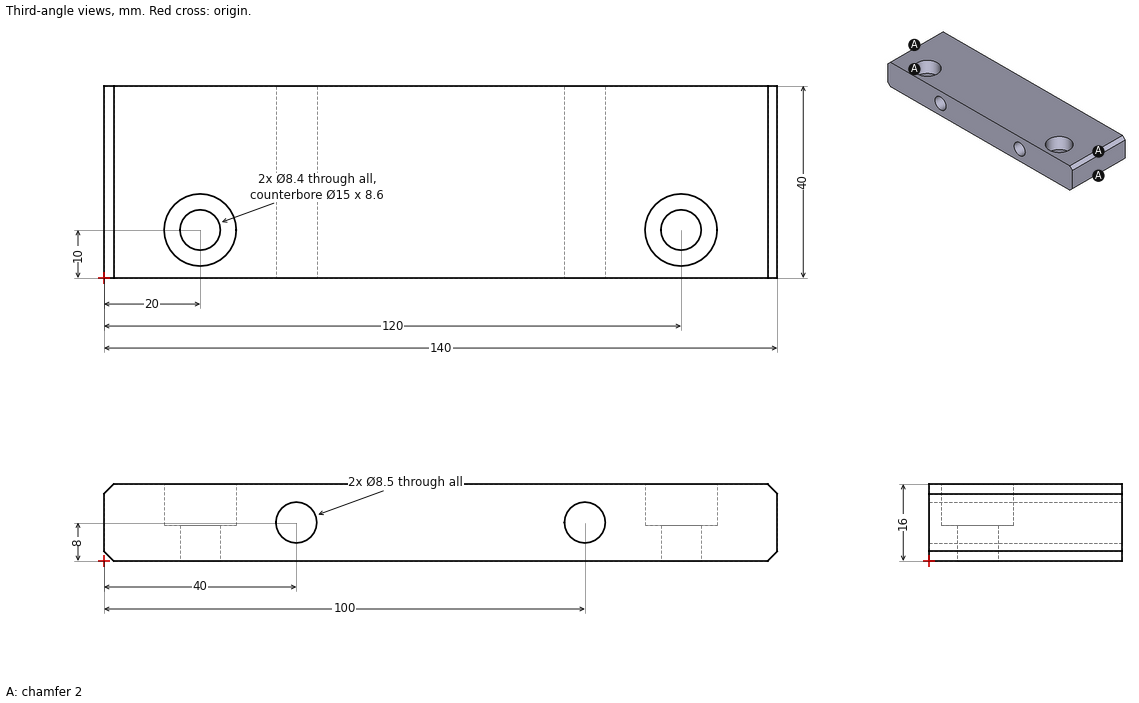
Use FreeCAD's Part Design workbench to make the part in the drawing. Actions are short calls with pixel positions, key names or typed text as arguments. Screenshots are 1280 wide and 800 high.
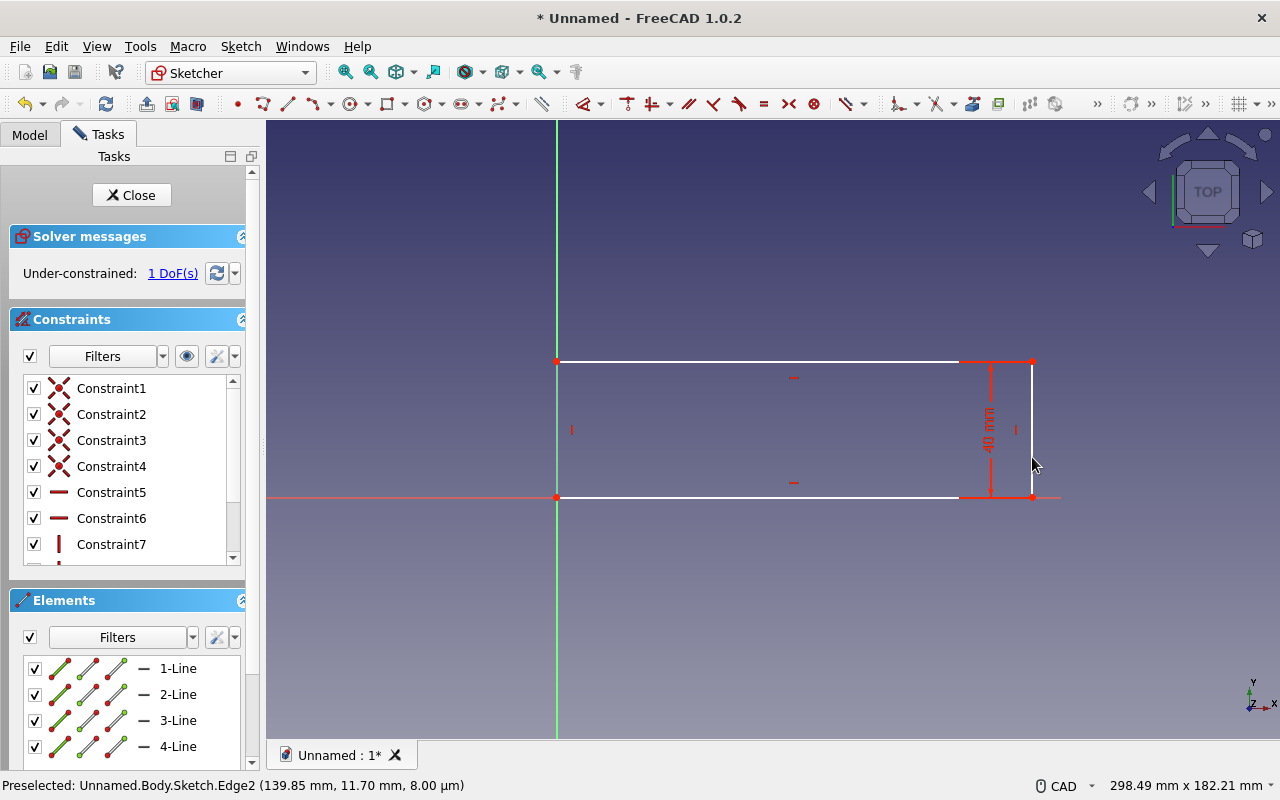
click(699, 498)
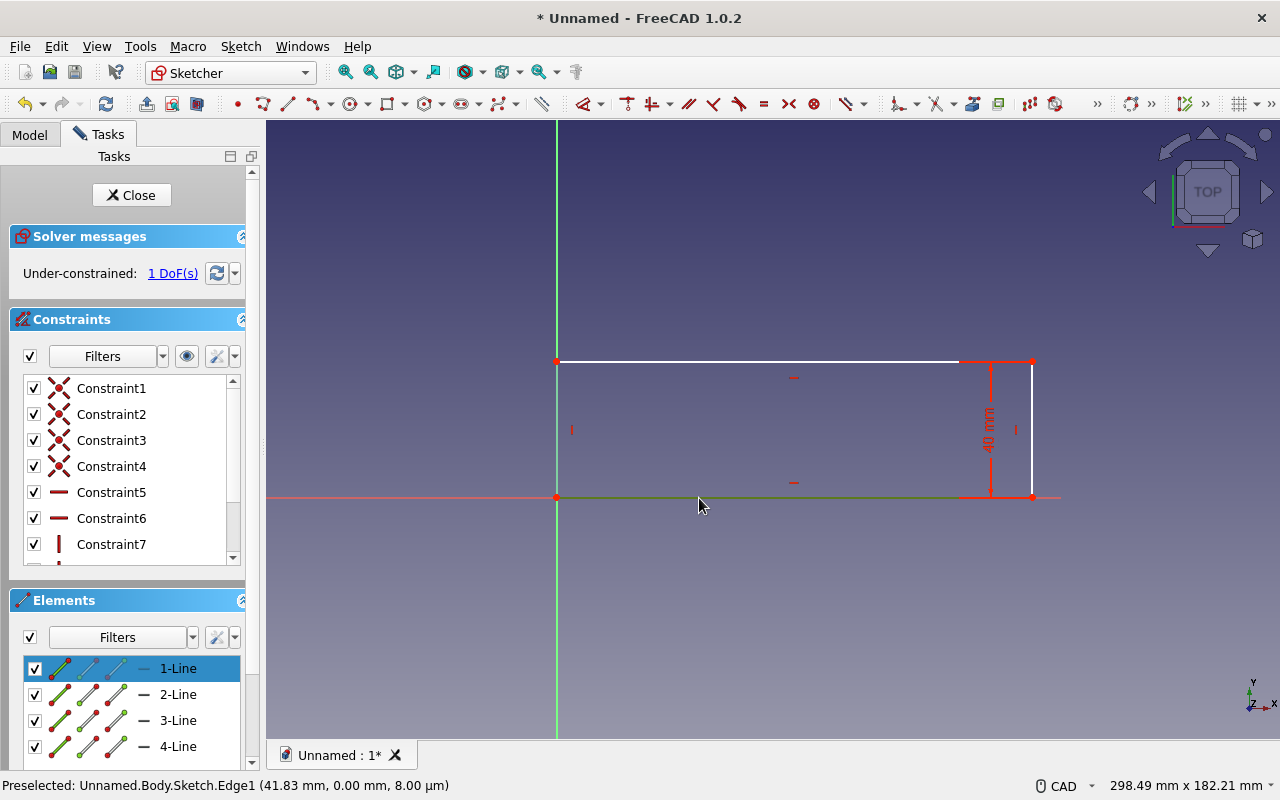
click(600, 104)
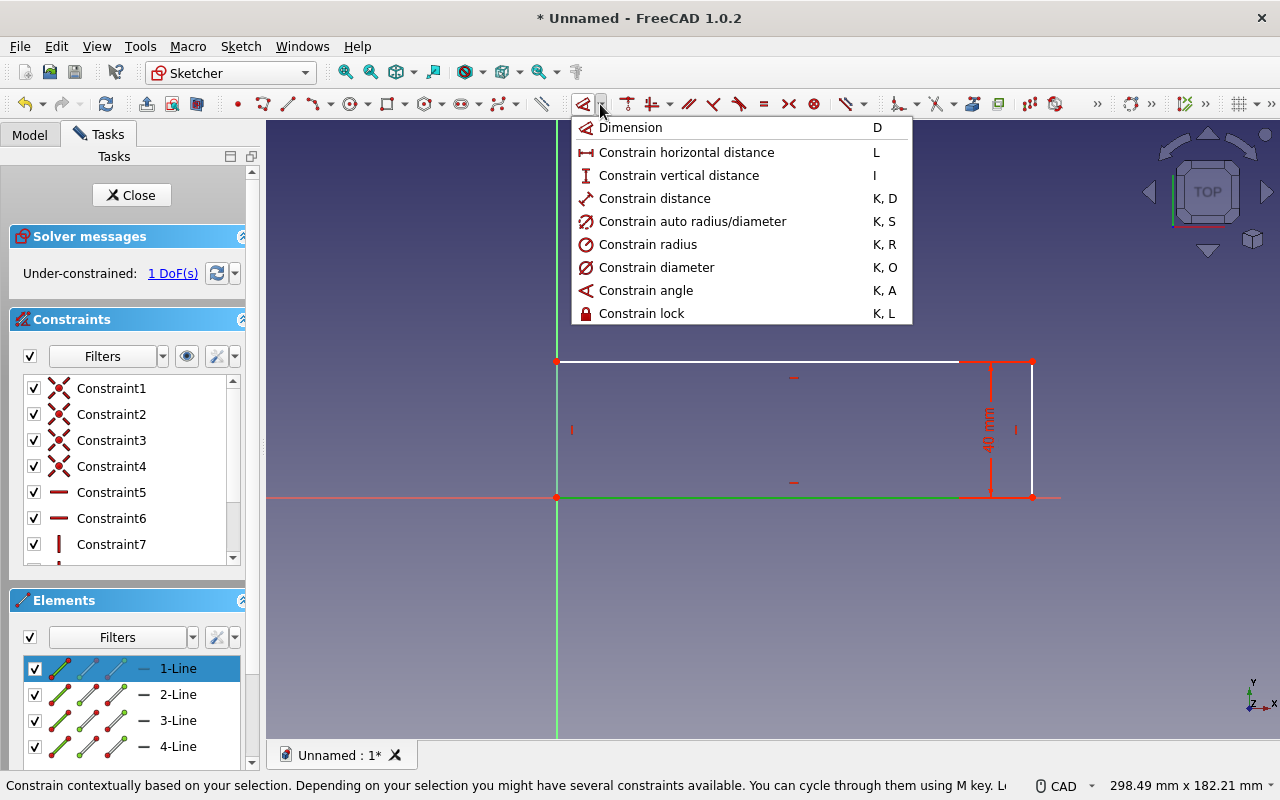
click(742, 152)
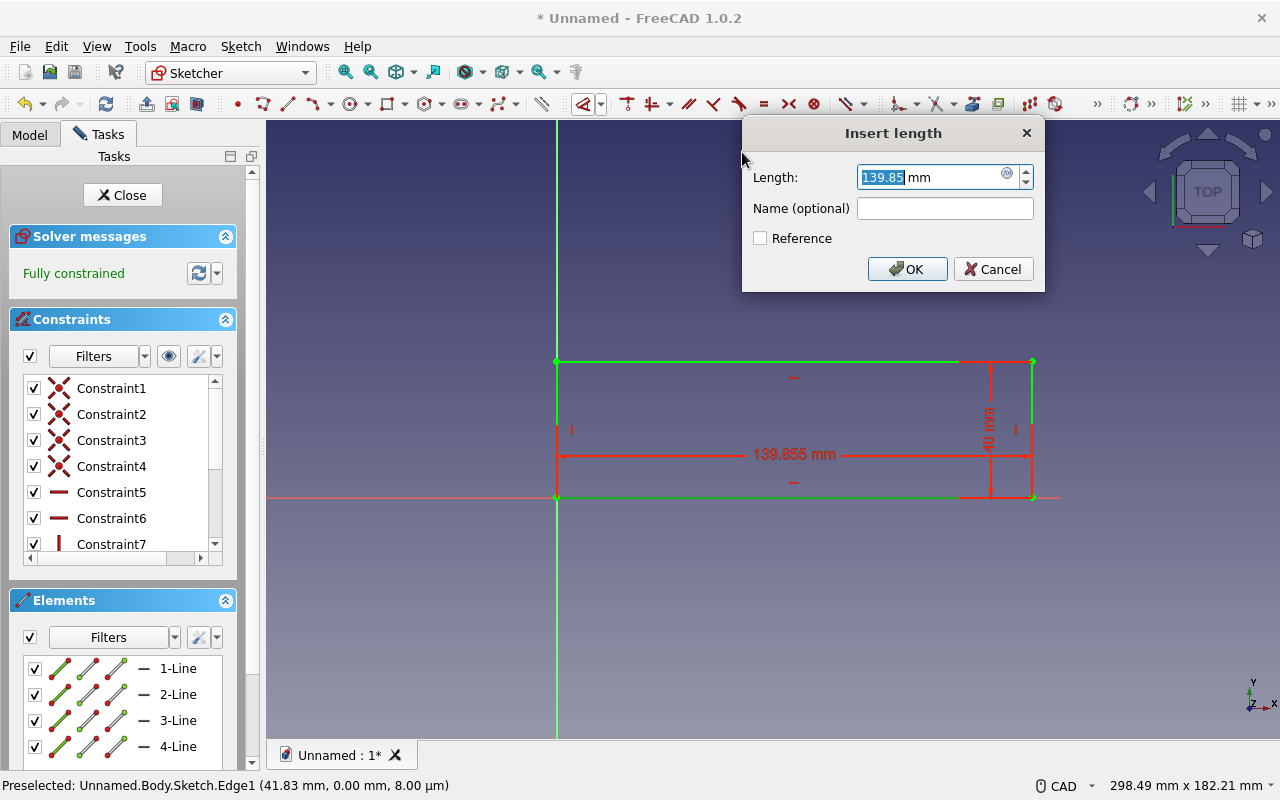
text(140)
key(Return)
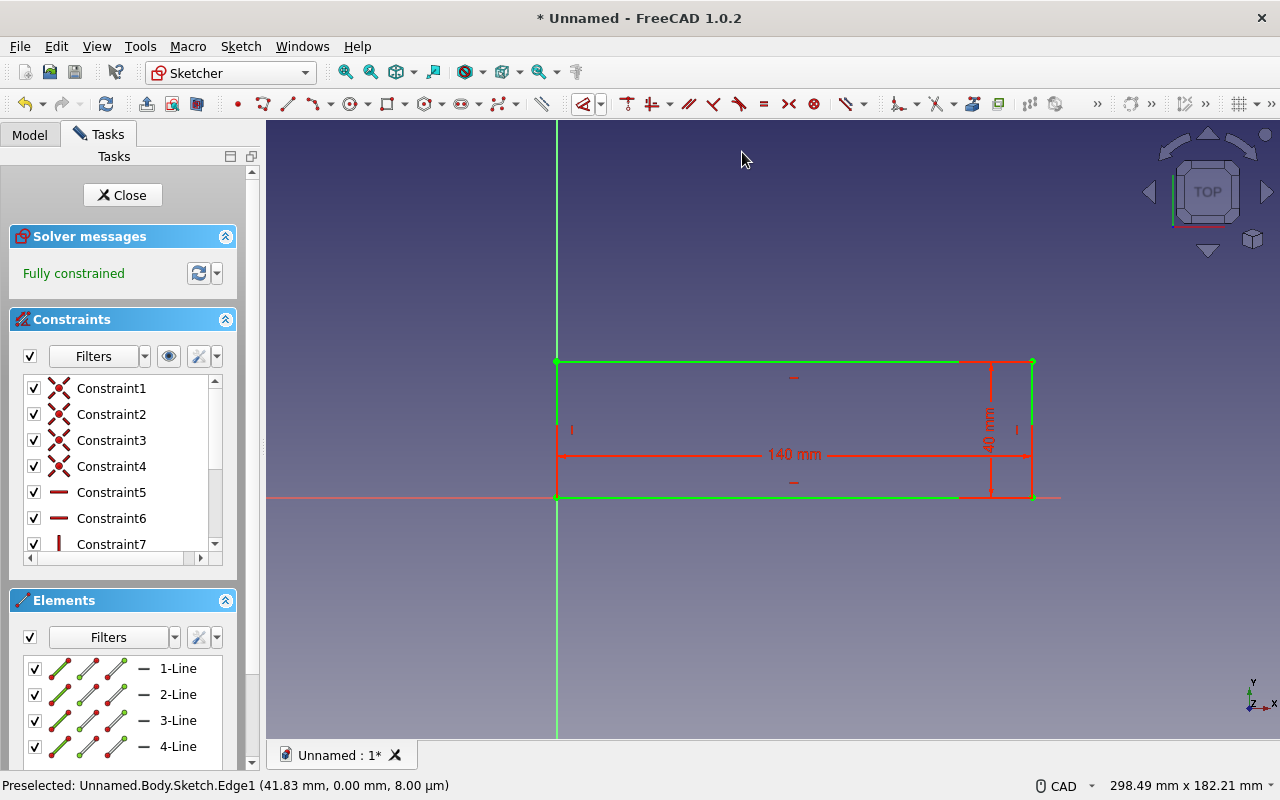
click(123, 195)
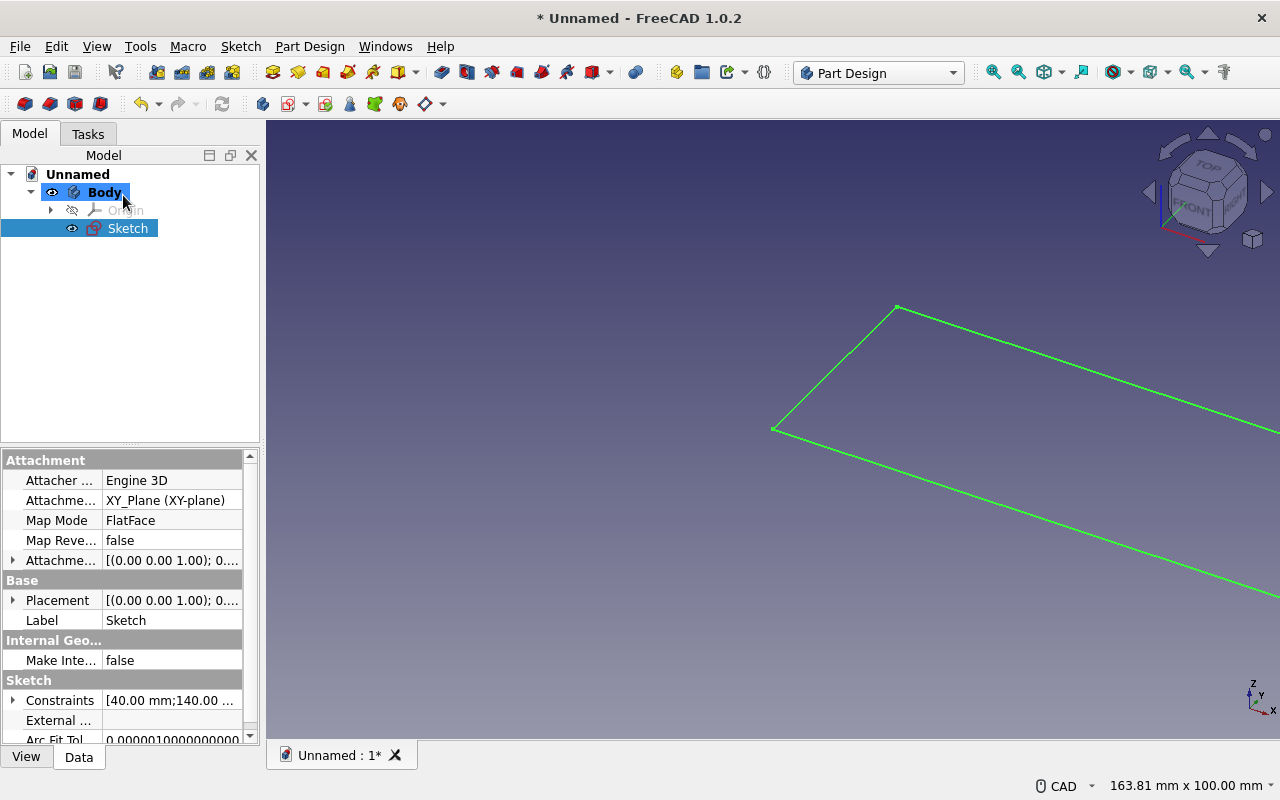
click(273, 72)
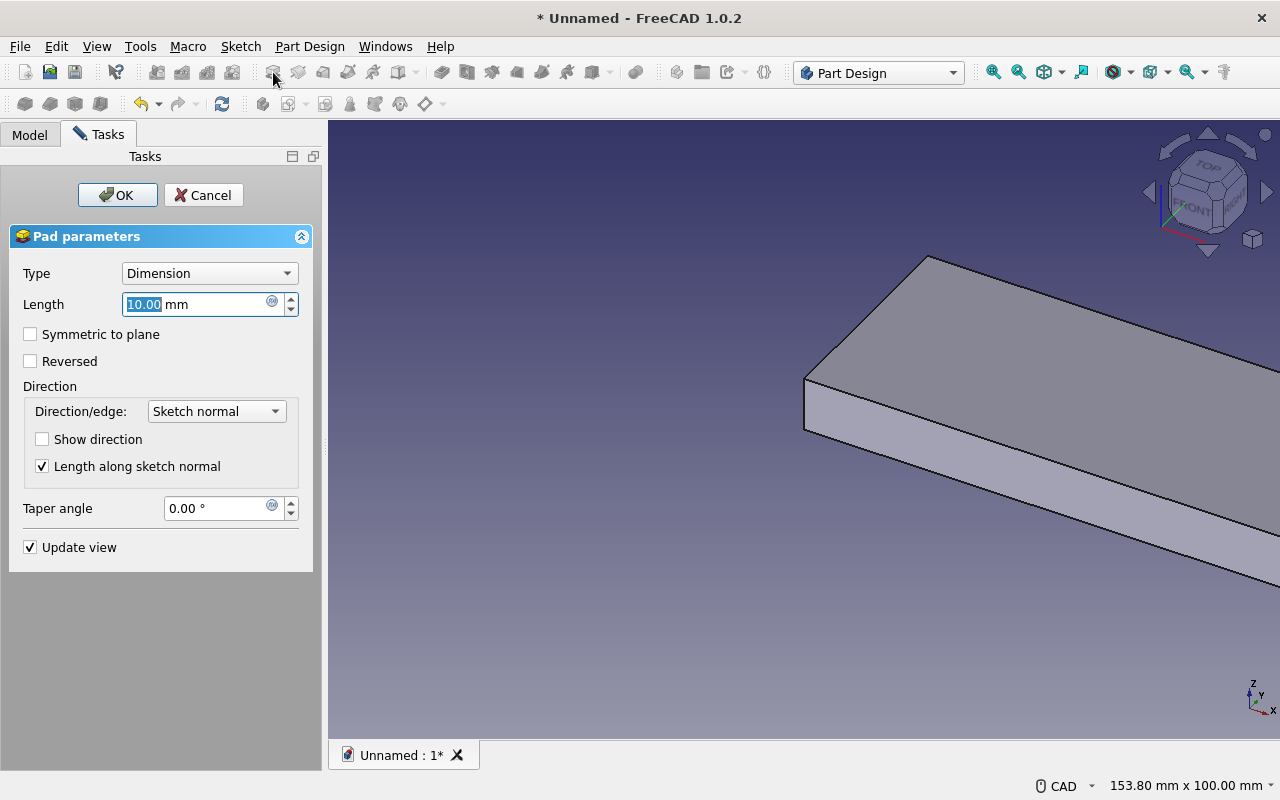
text(16)
key(Tab)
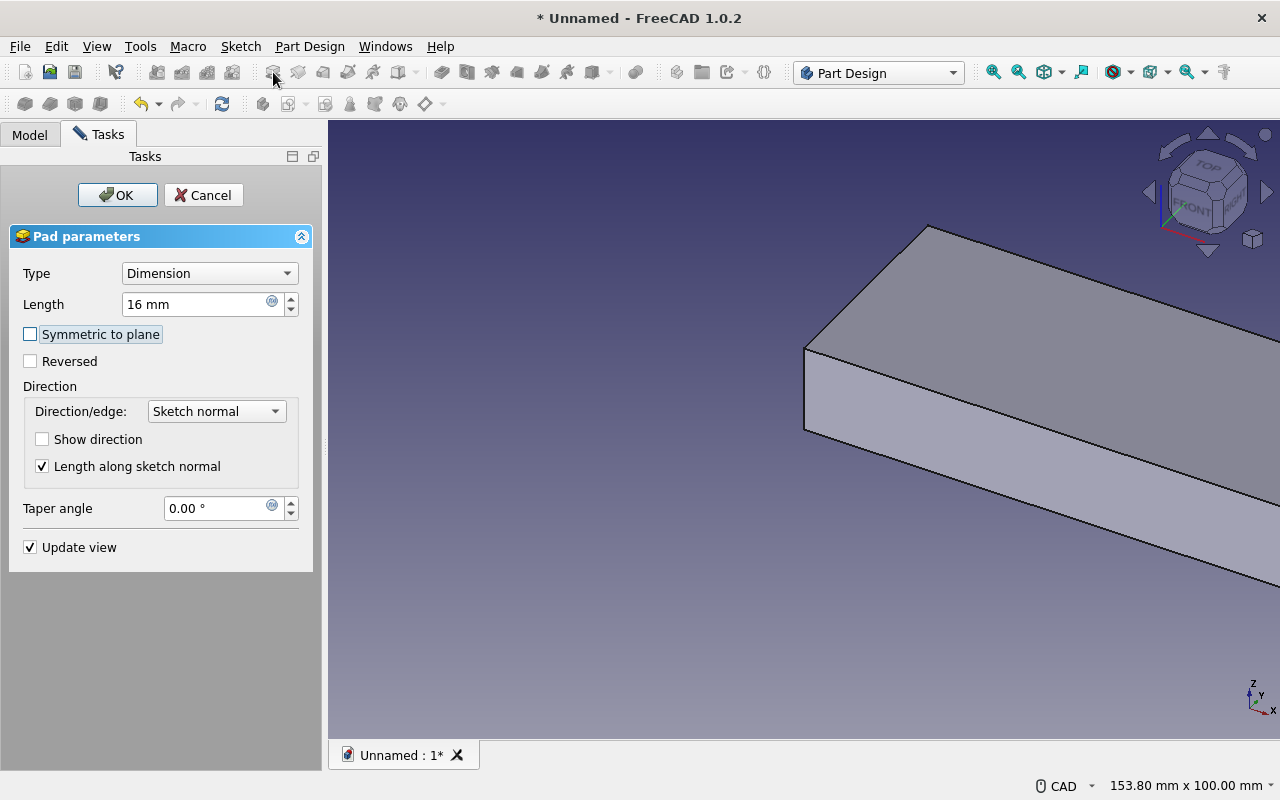
click(118, 195)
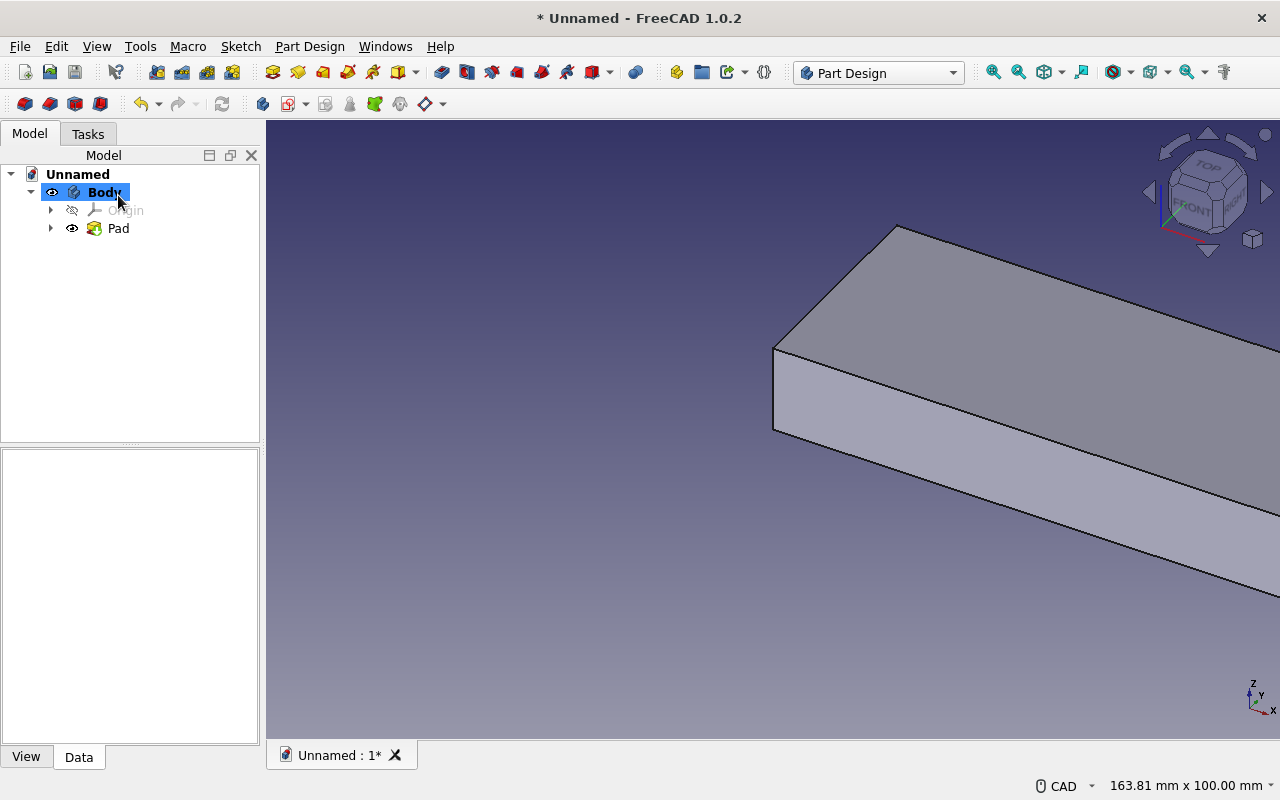
click(994, 72)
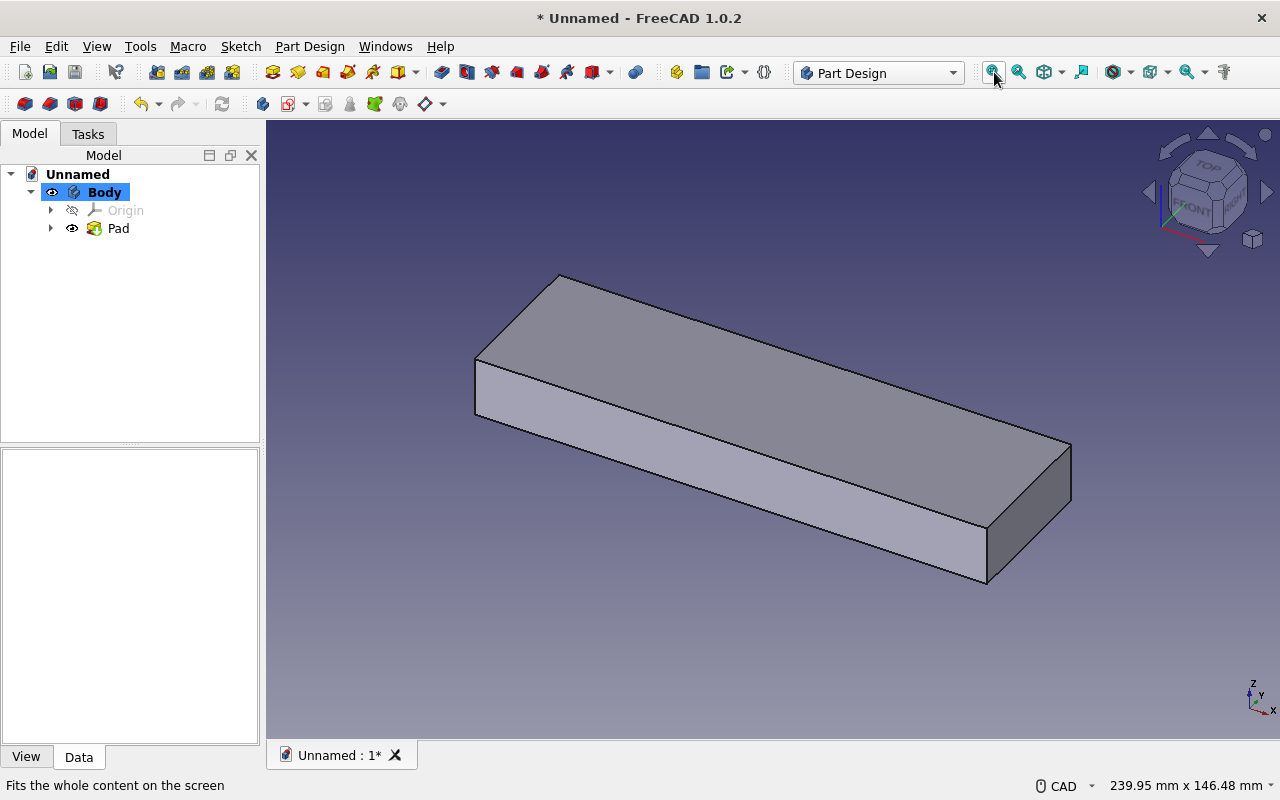
key(4)